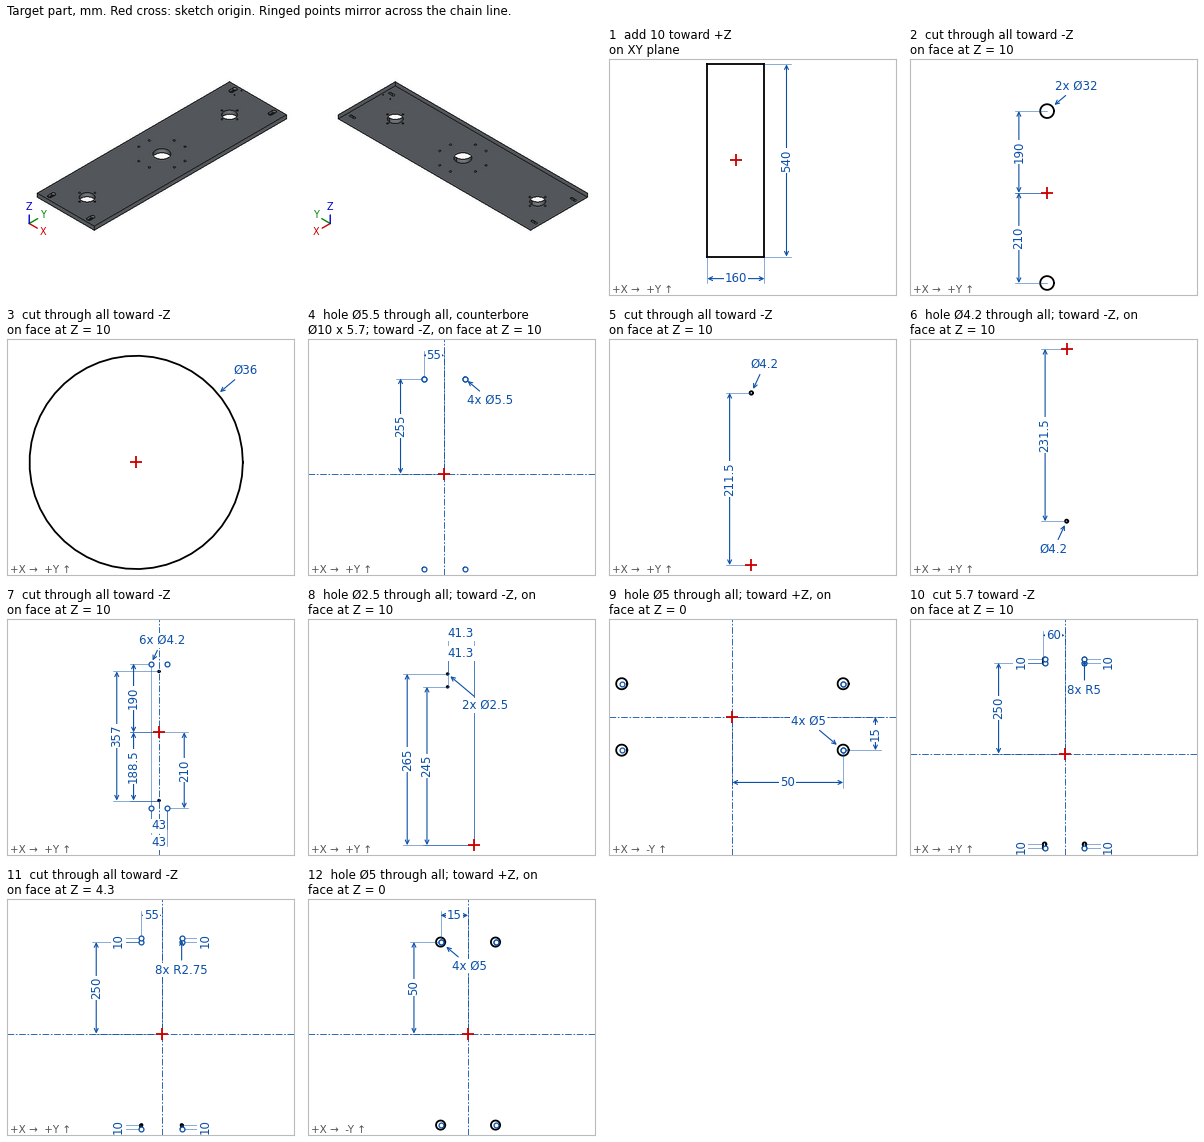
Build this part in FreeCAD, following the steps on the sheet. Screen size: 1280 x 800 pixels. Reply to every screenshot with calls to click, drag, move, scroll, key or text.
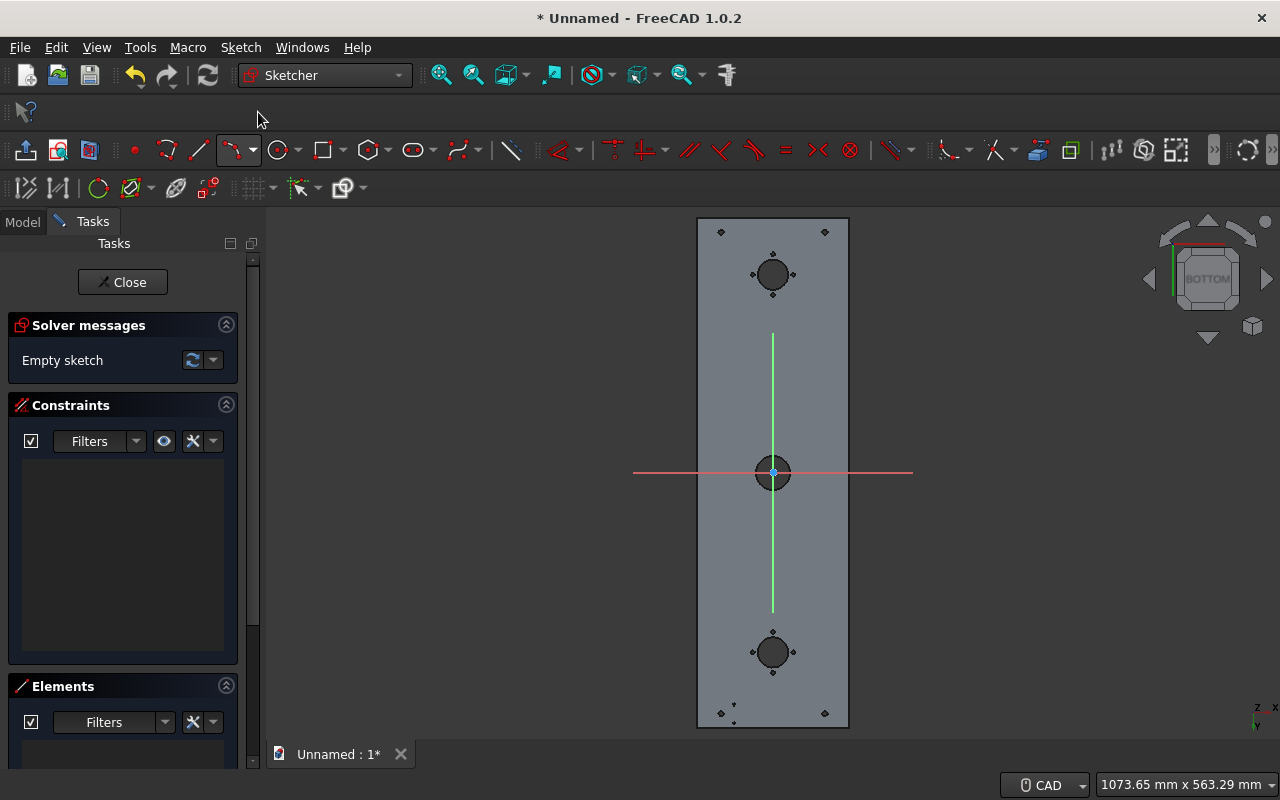
scroll(787, 473, up, 9)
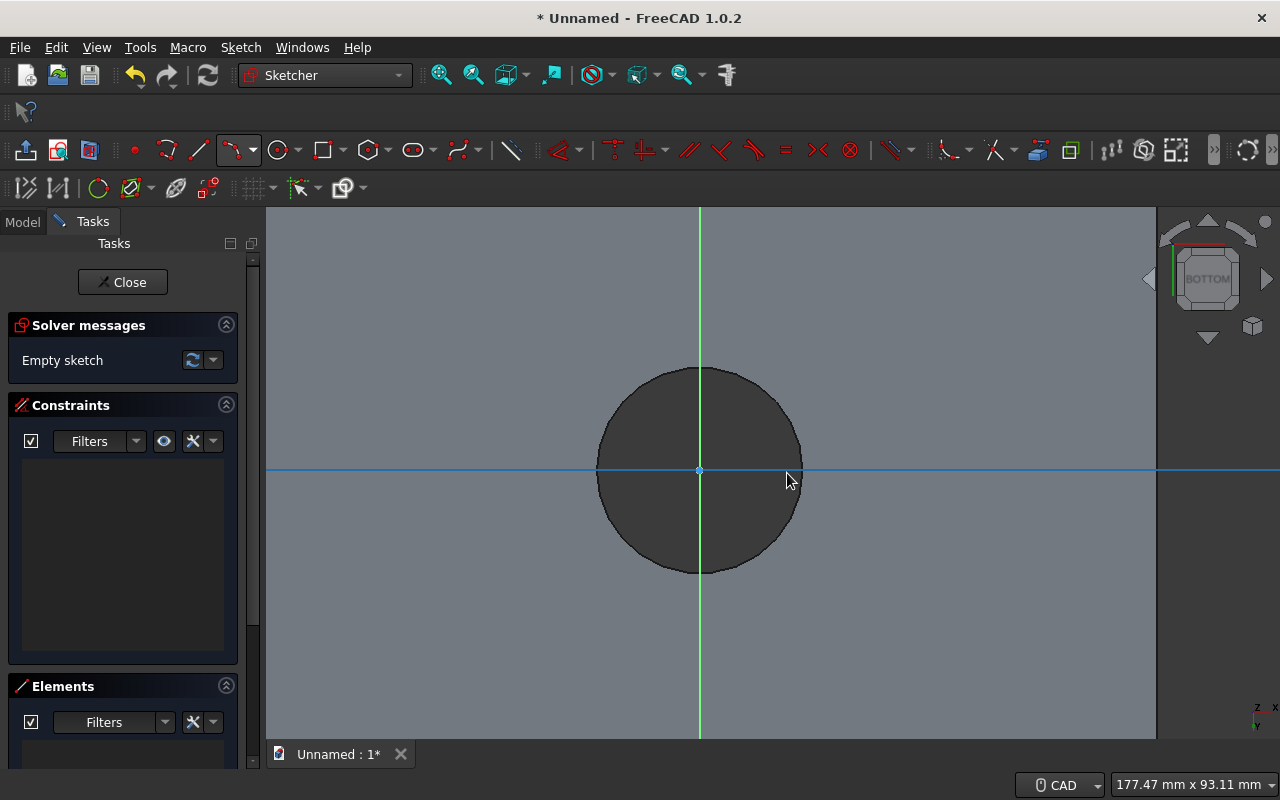
key(g)
key(c)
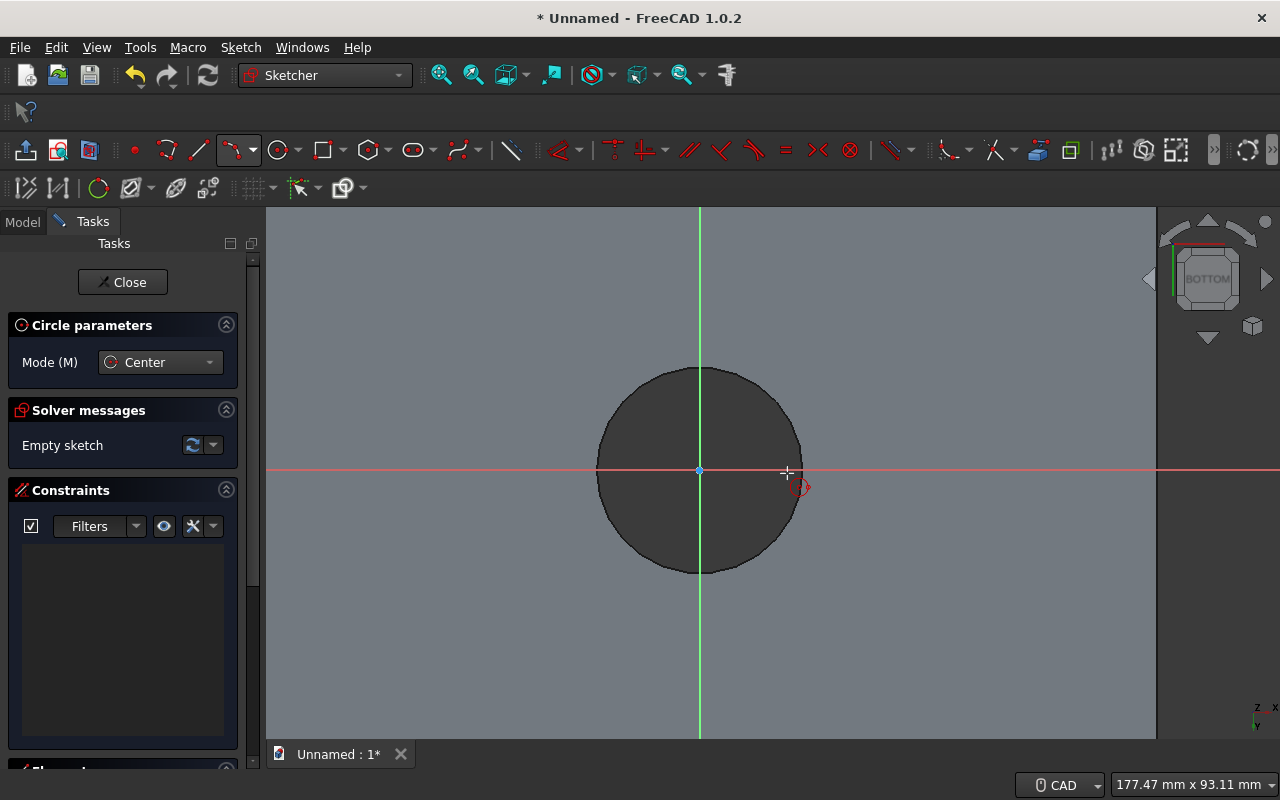
scroll(985, 556, up, 3)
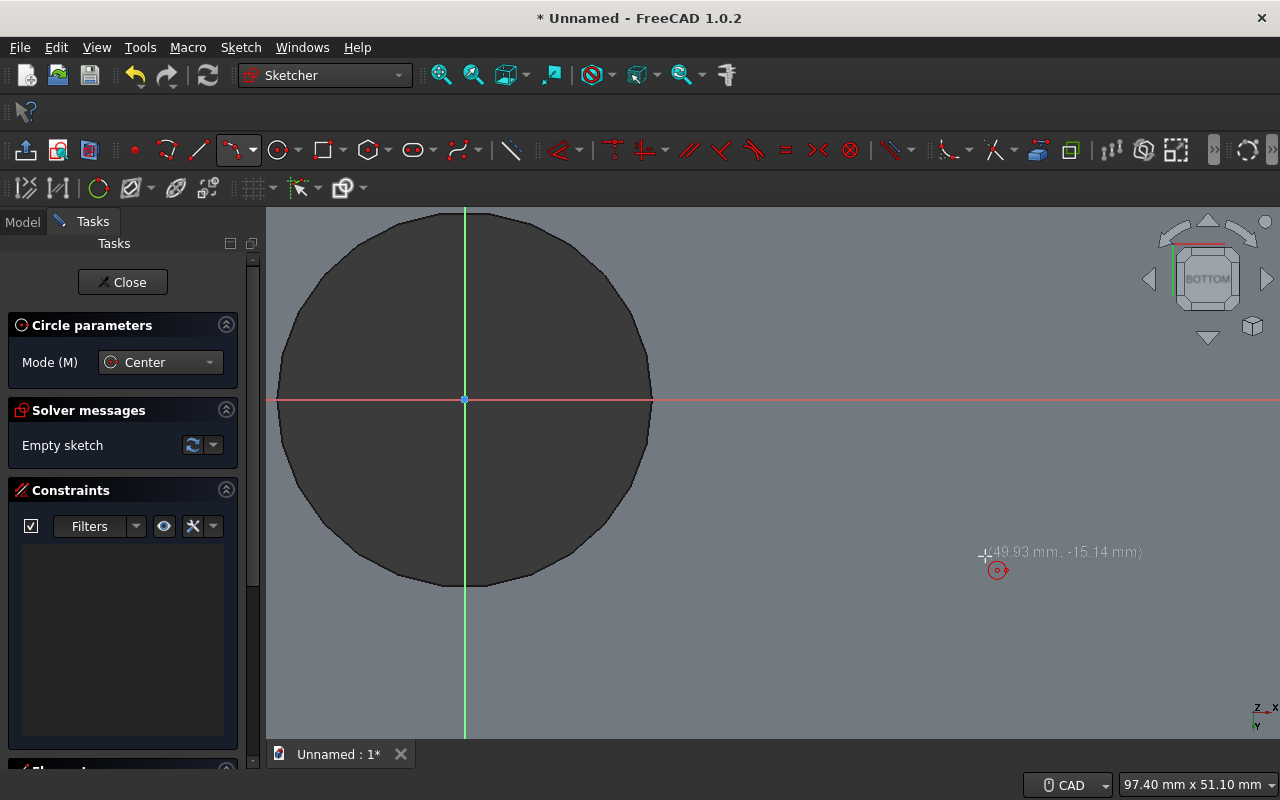
click(985, 556)
move(1004, 537)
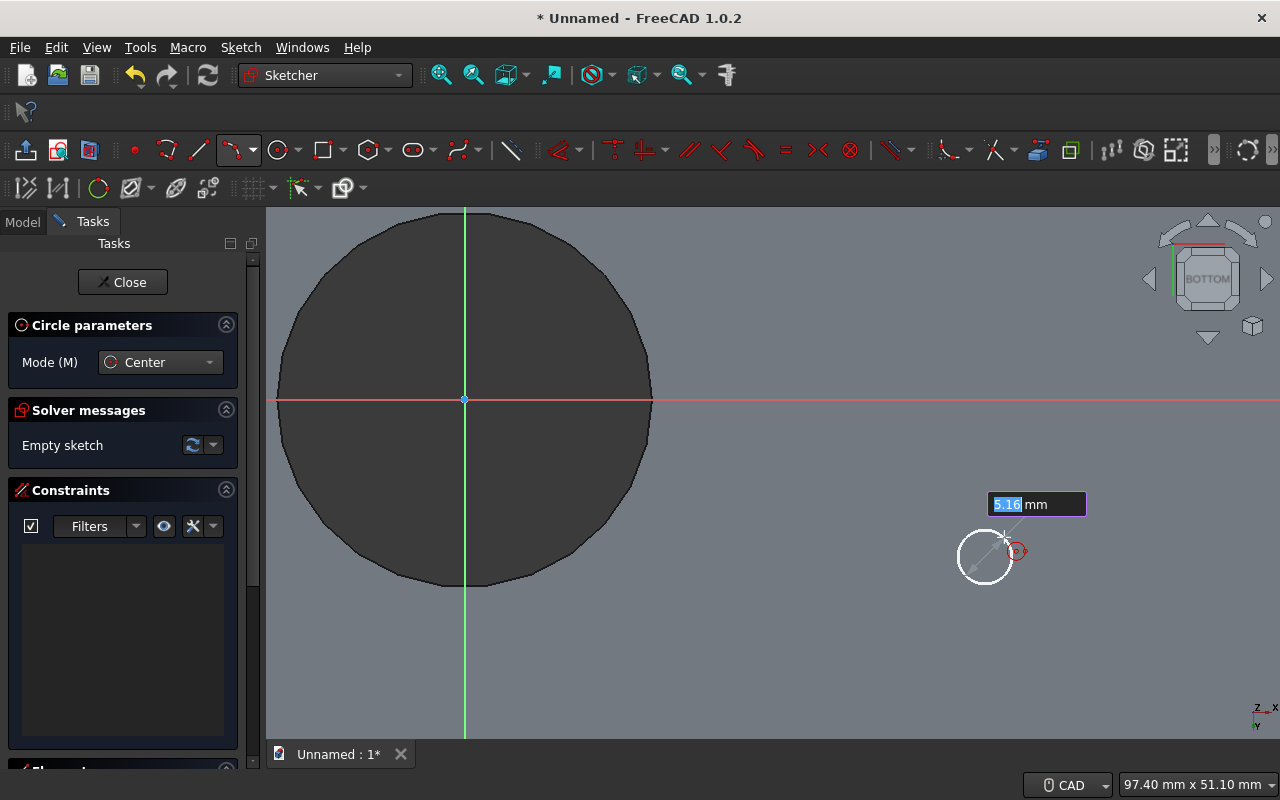
text(5)
key(Return)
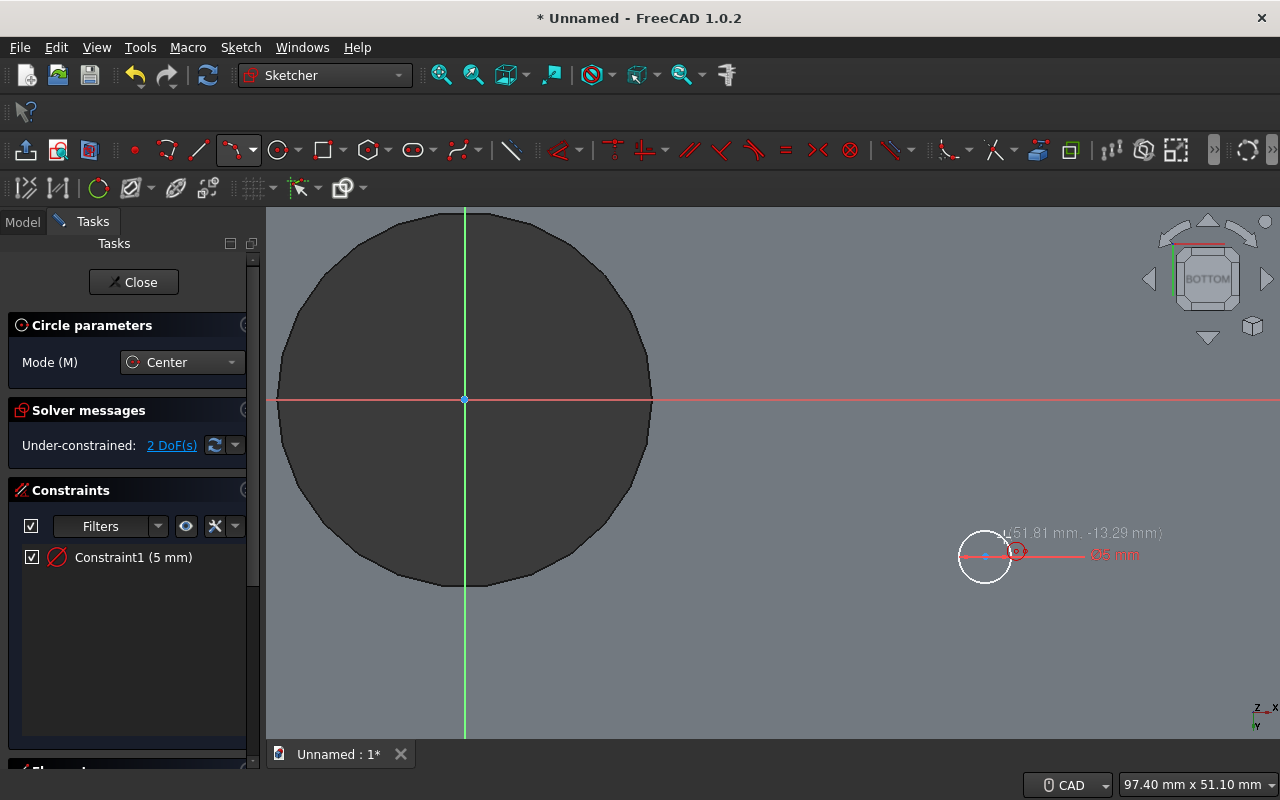
click(985, 243)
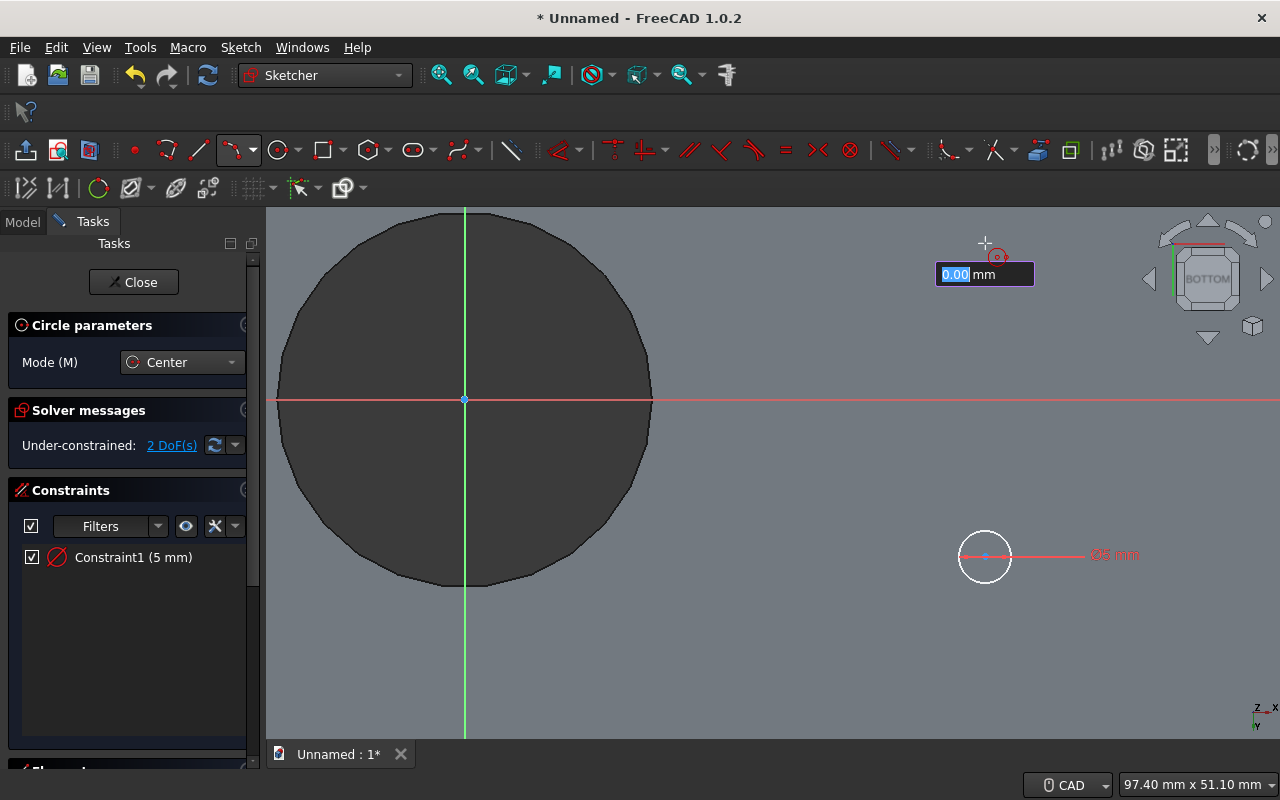
scroll(996, 562, down, 3)
move(1000, 377)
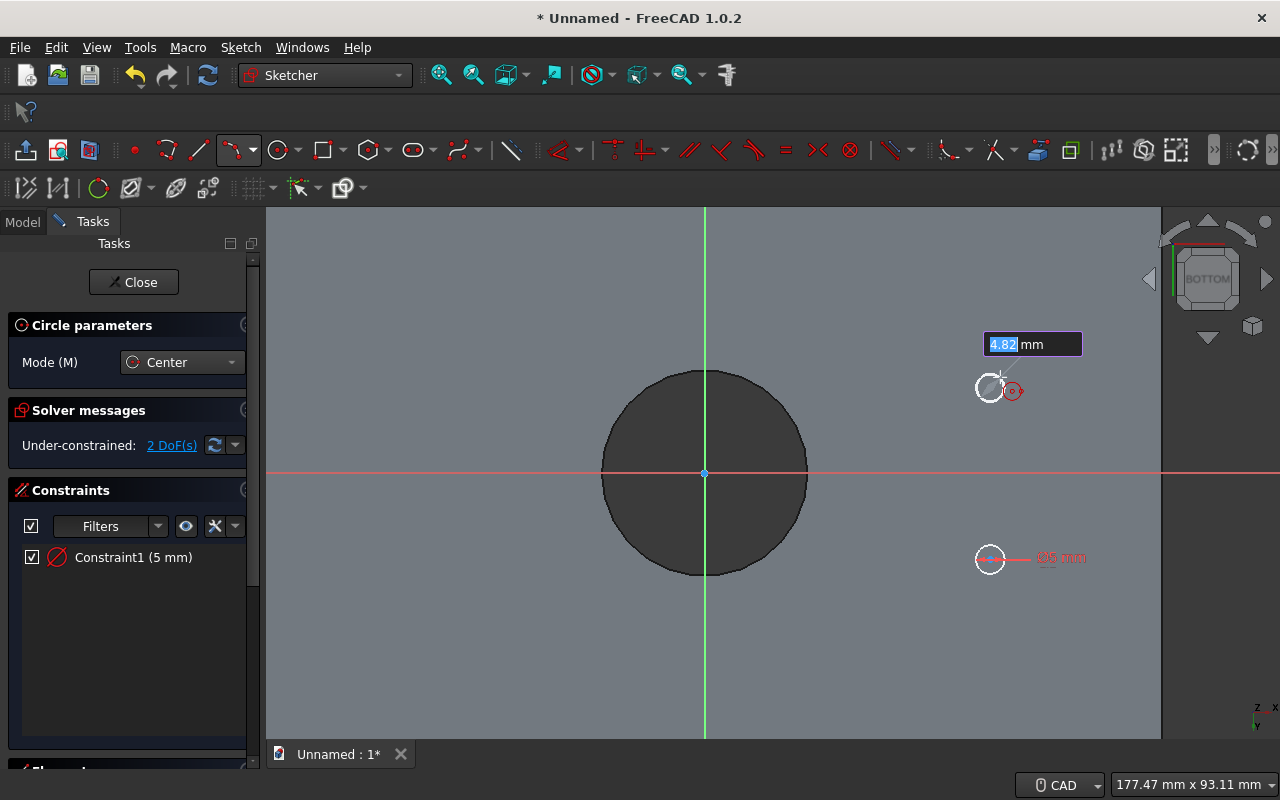
text(5)
key(Return)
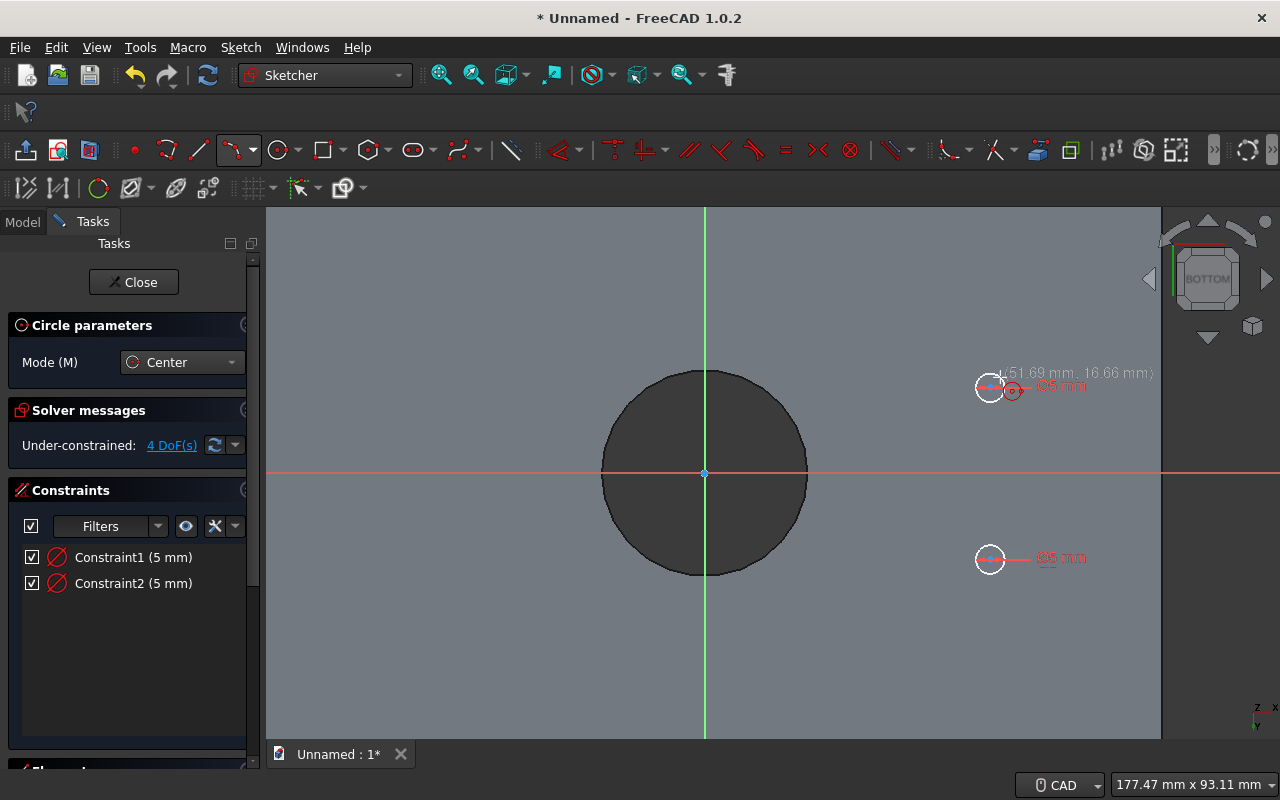
scroll(419, 559, up, 3)